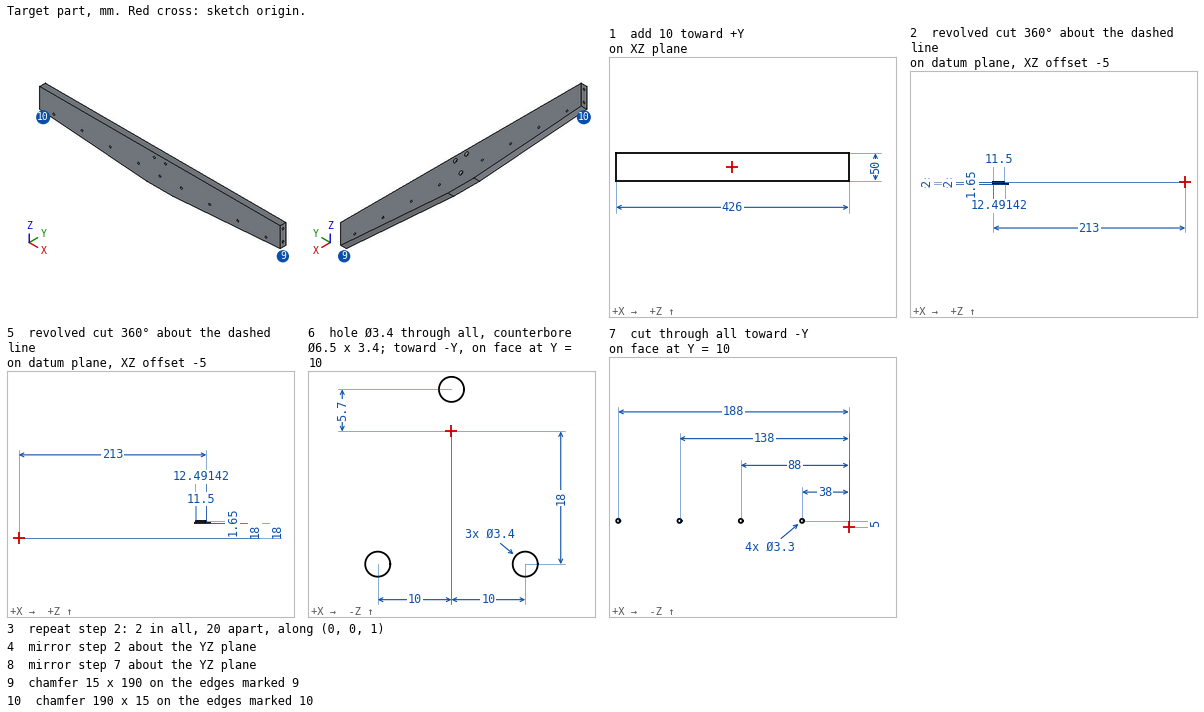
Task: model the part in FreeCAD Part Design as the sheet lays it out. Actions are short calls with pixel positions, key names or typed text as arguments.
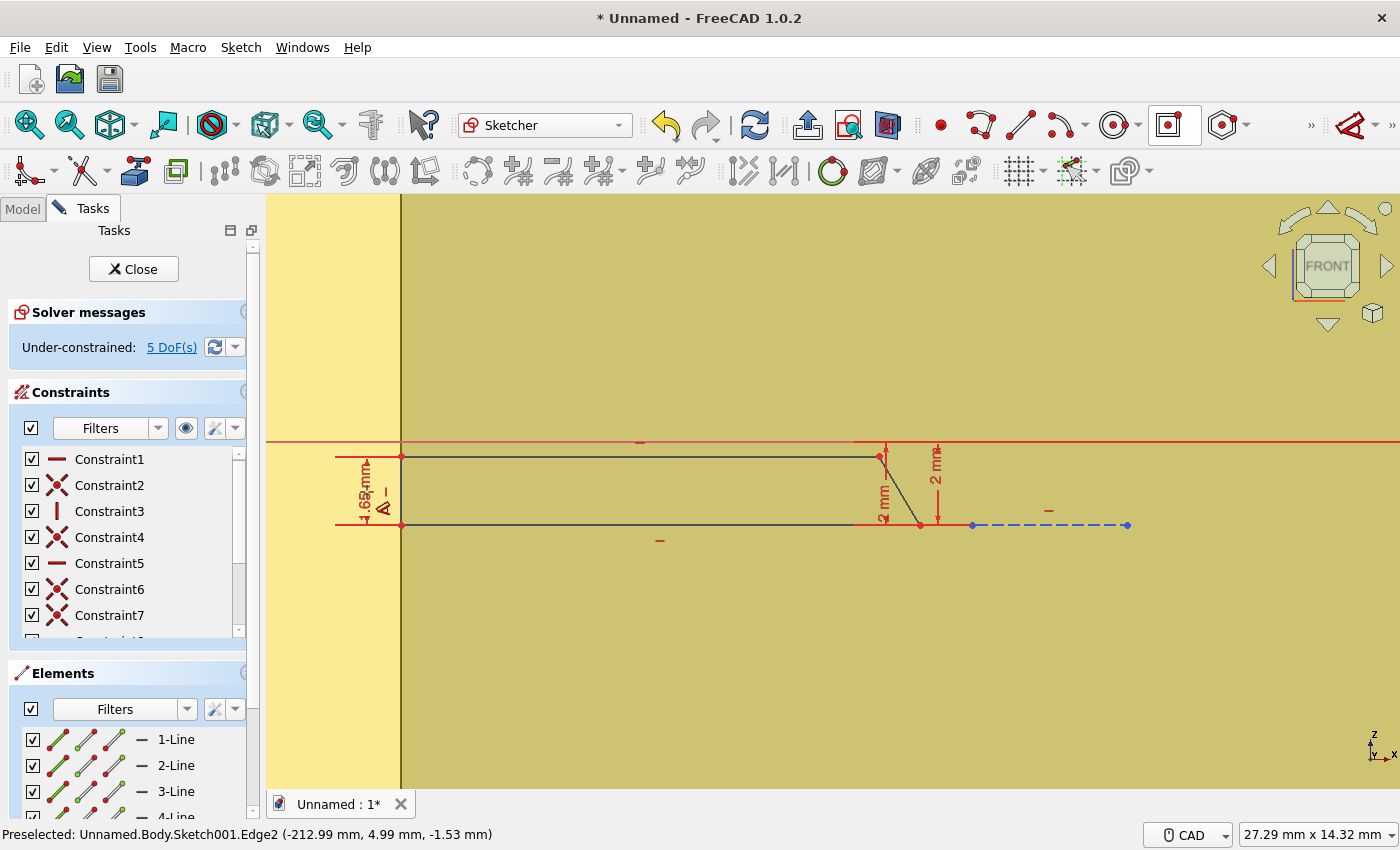
click(544, 457)
click(640, 423)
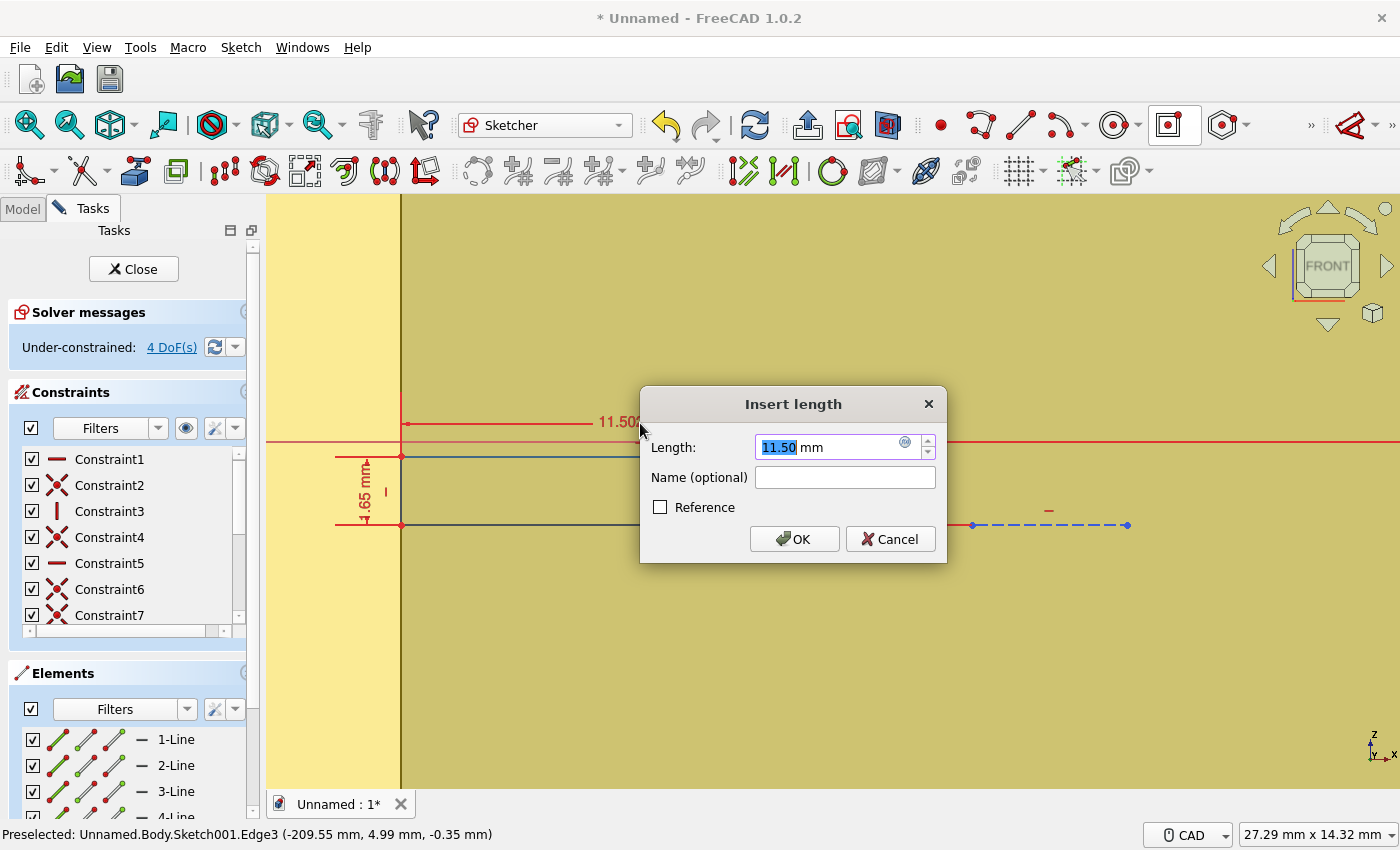
text(11.5)
key(Return)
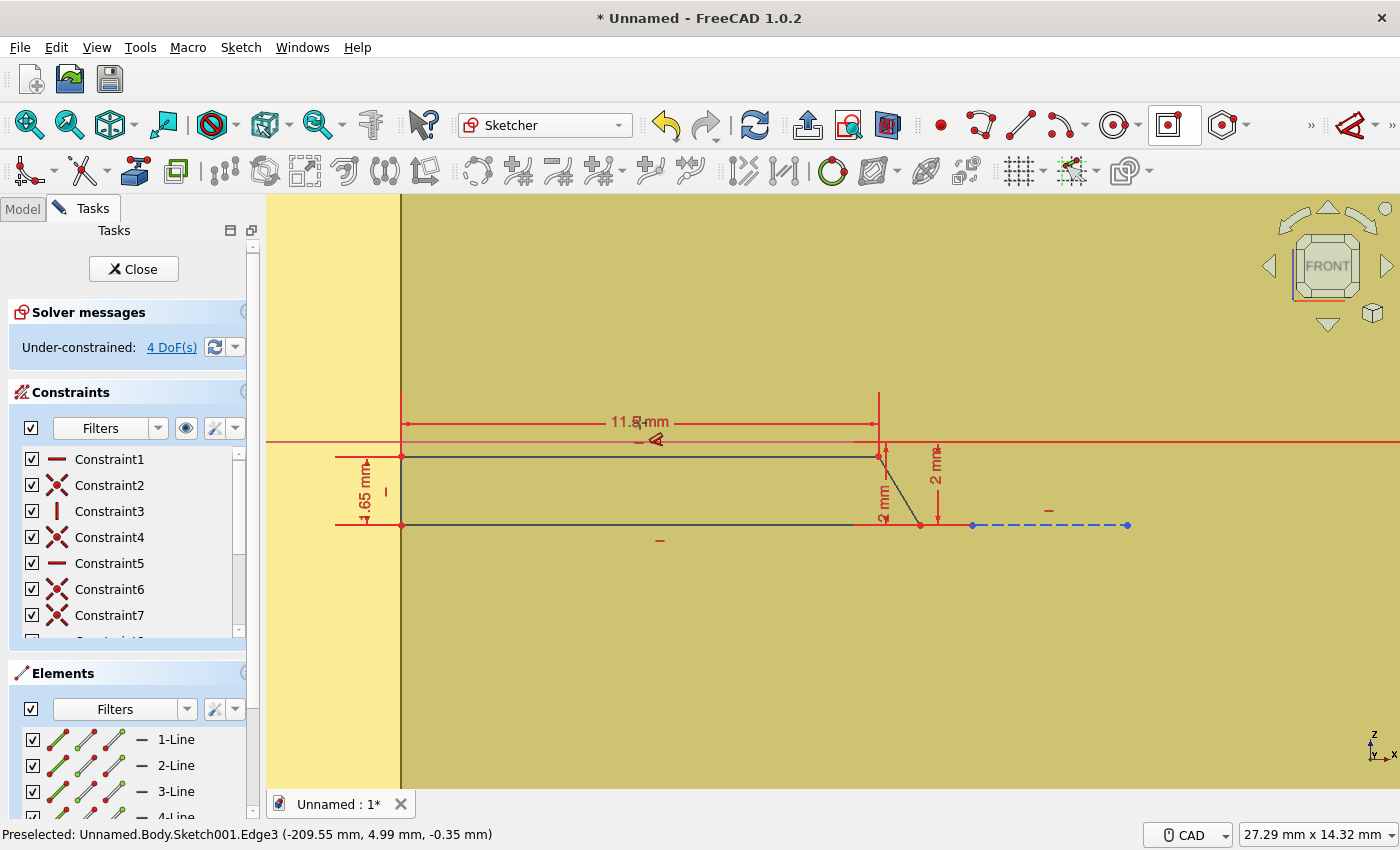
click(401, 525)
click(818, 408)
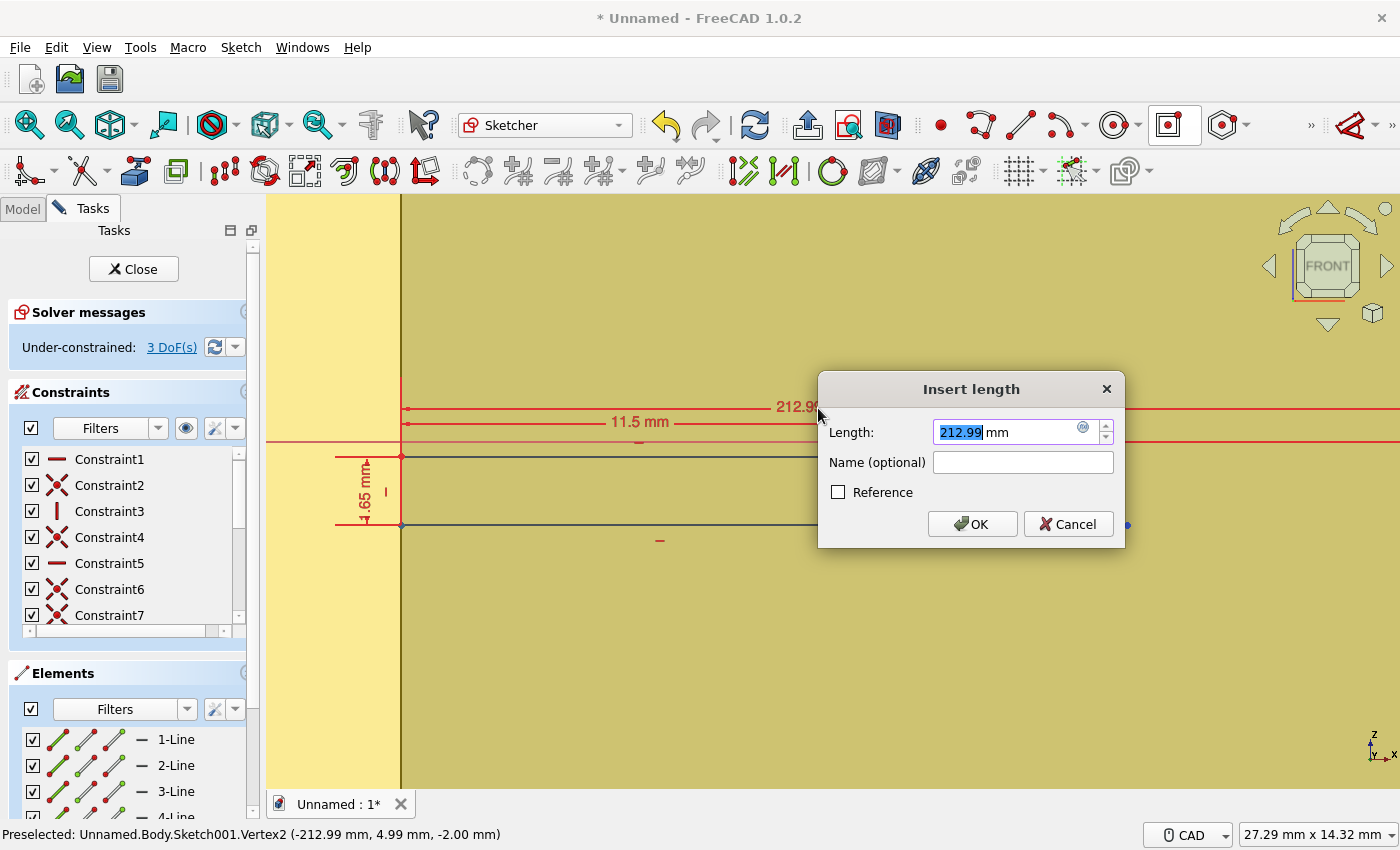
text(213)
key(Return)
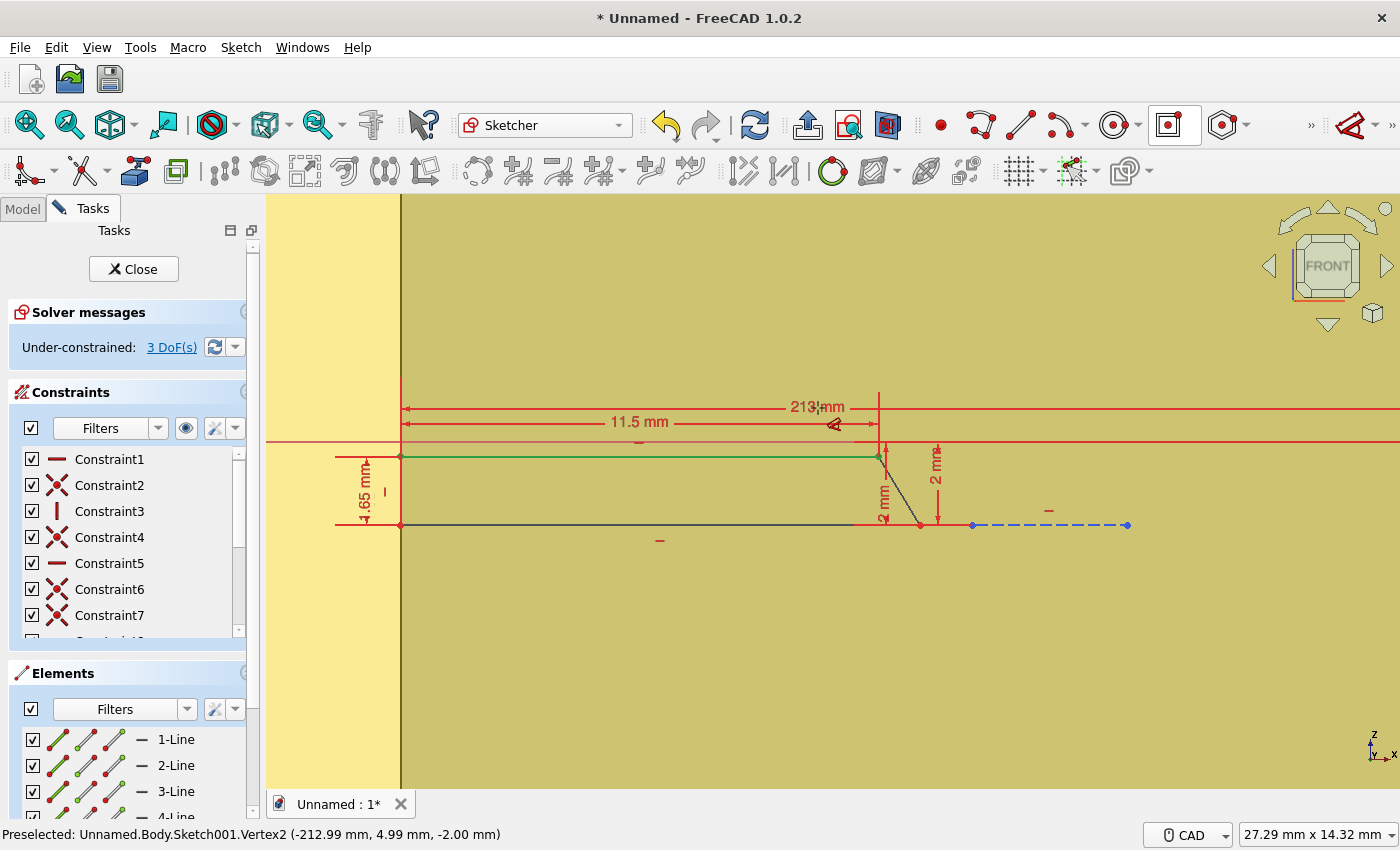
click(764, 525)
click(660, 559)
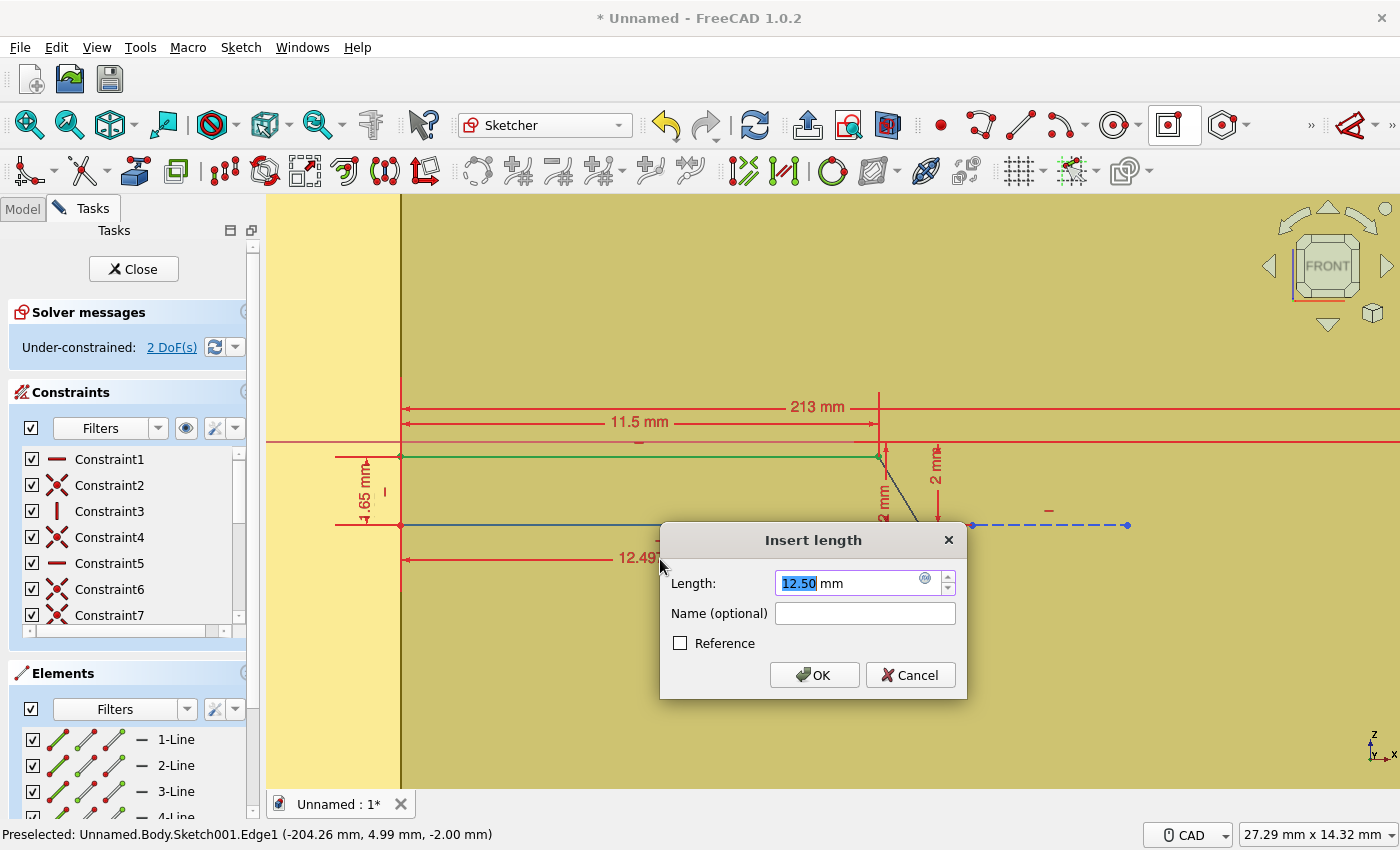
text(12.49142)
key(Return)
key(Escape)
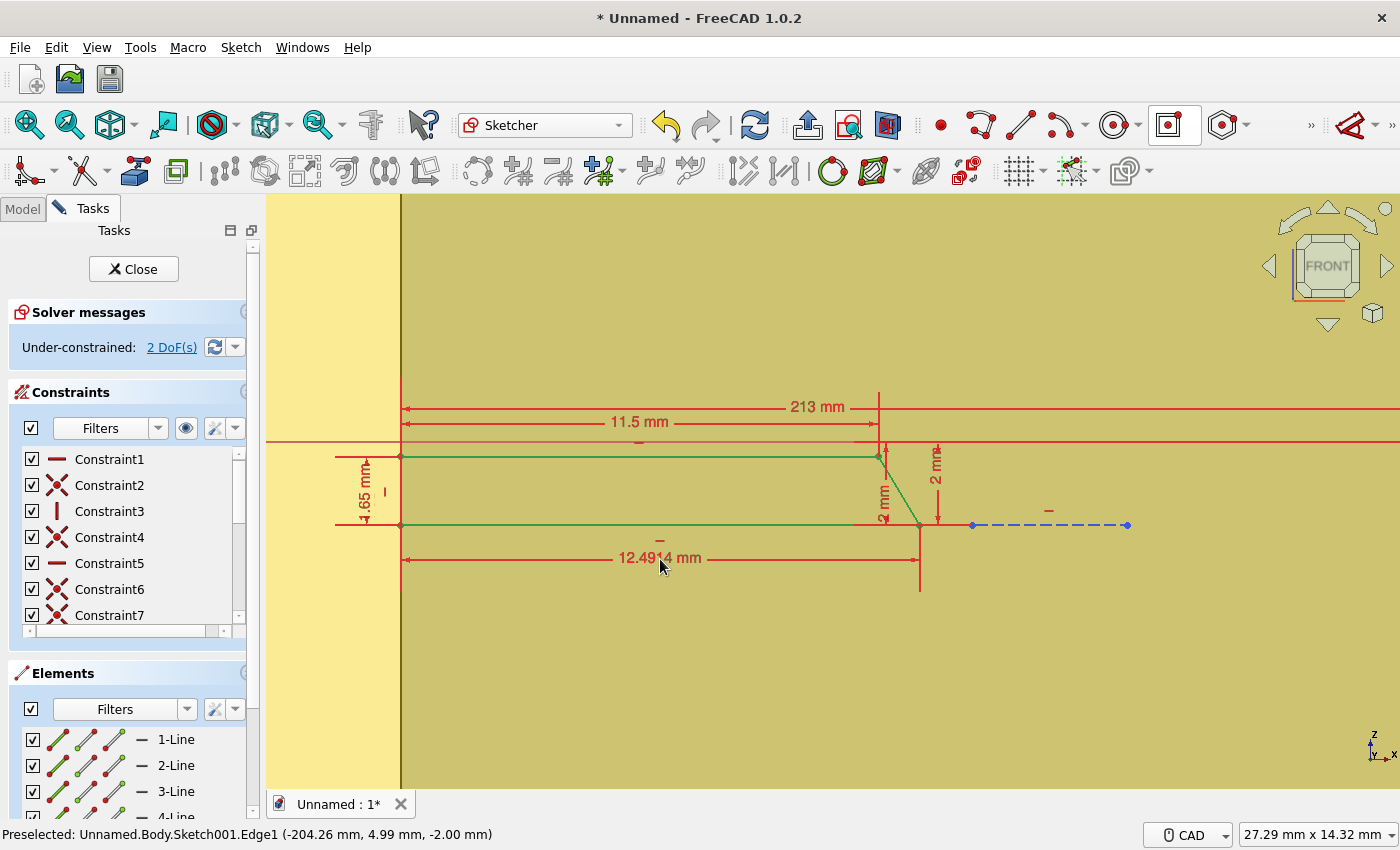
click(134, 269)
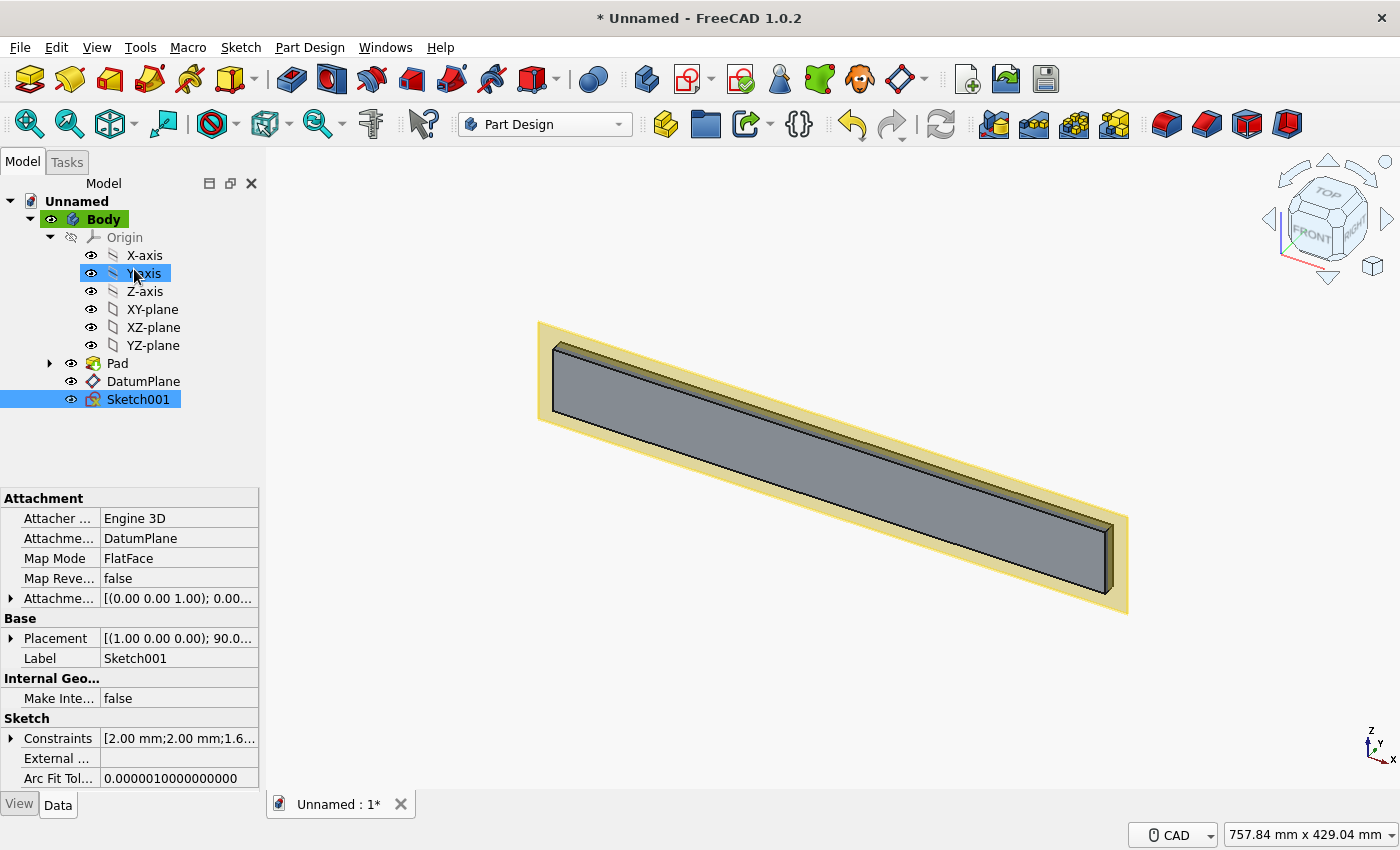
click(372, 80)